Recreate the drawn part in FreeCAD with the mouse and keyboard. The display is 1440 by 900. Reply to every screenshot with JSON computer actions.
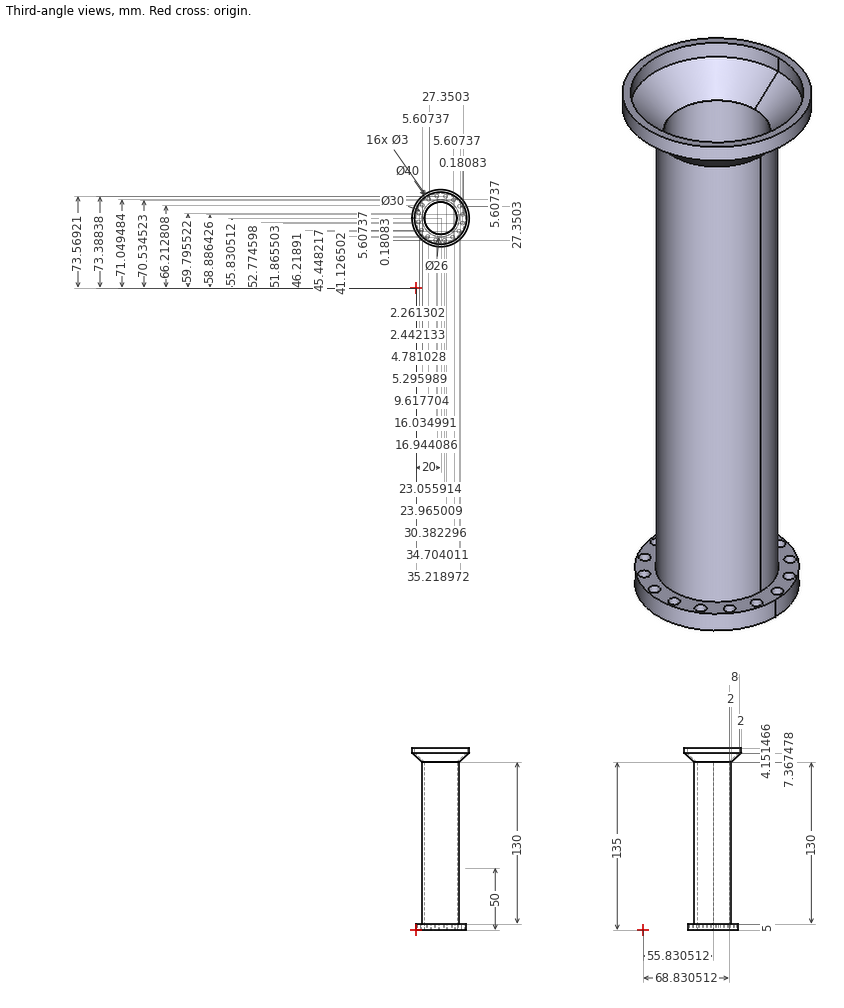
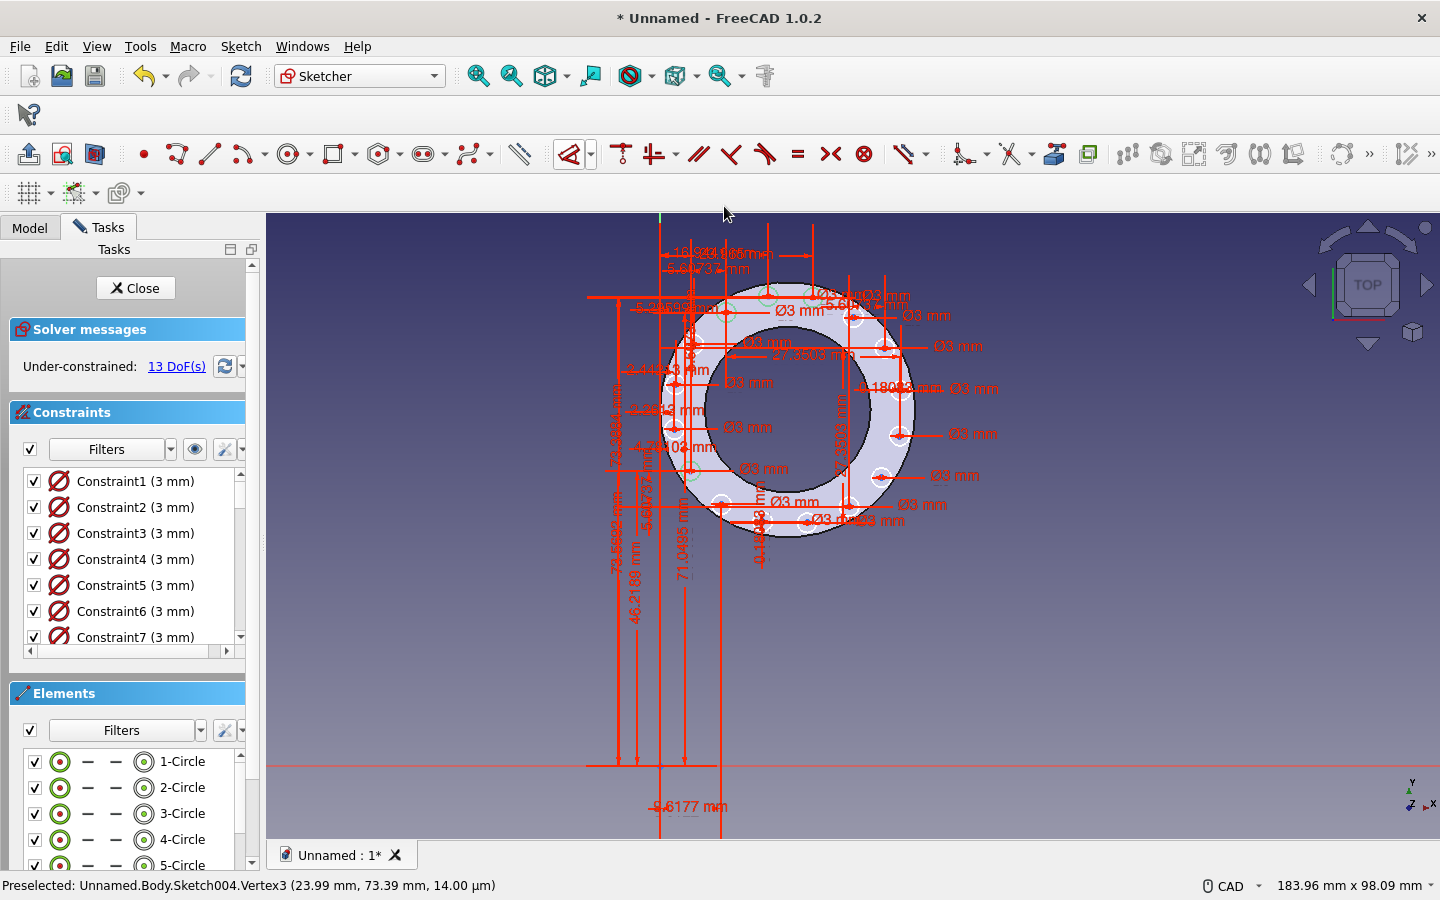
{"action": "left_click", "coordinate": [853, 318]}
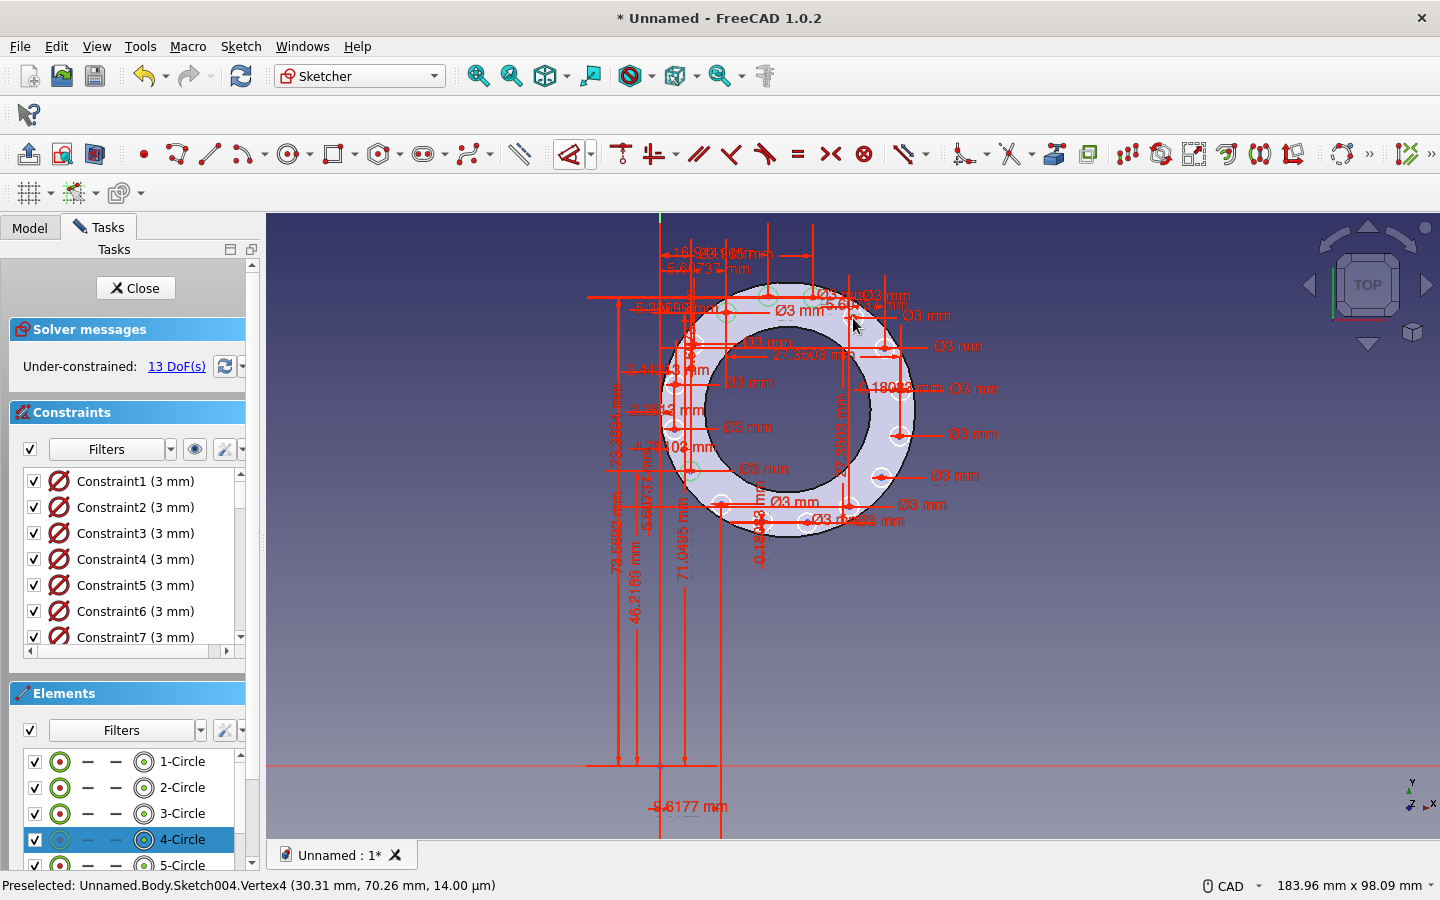
{"action": "key", "text": "l"}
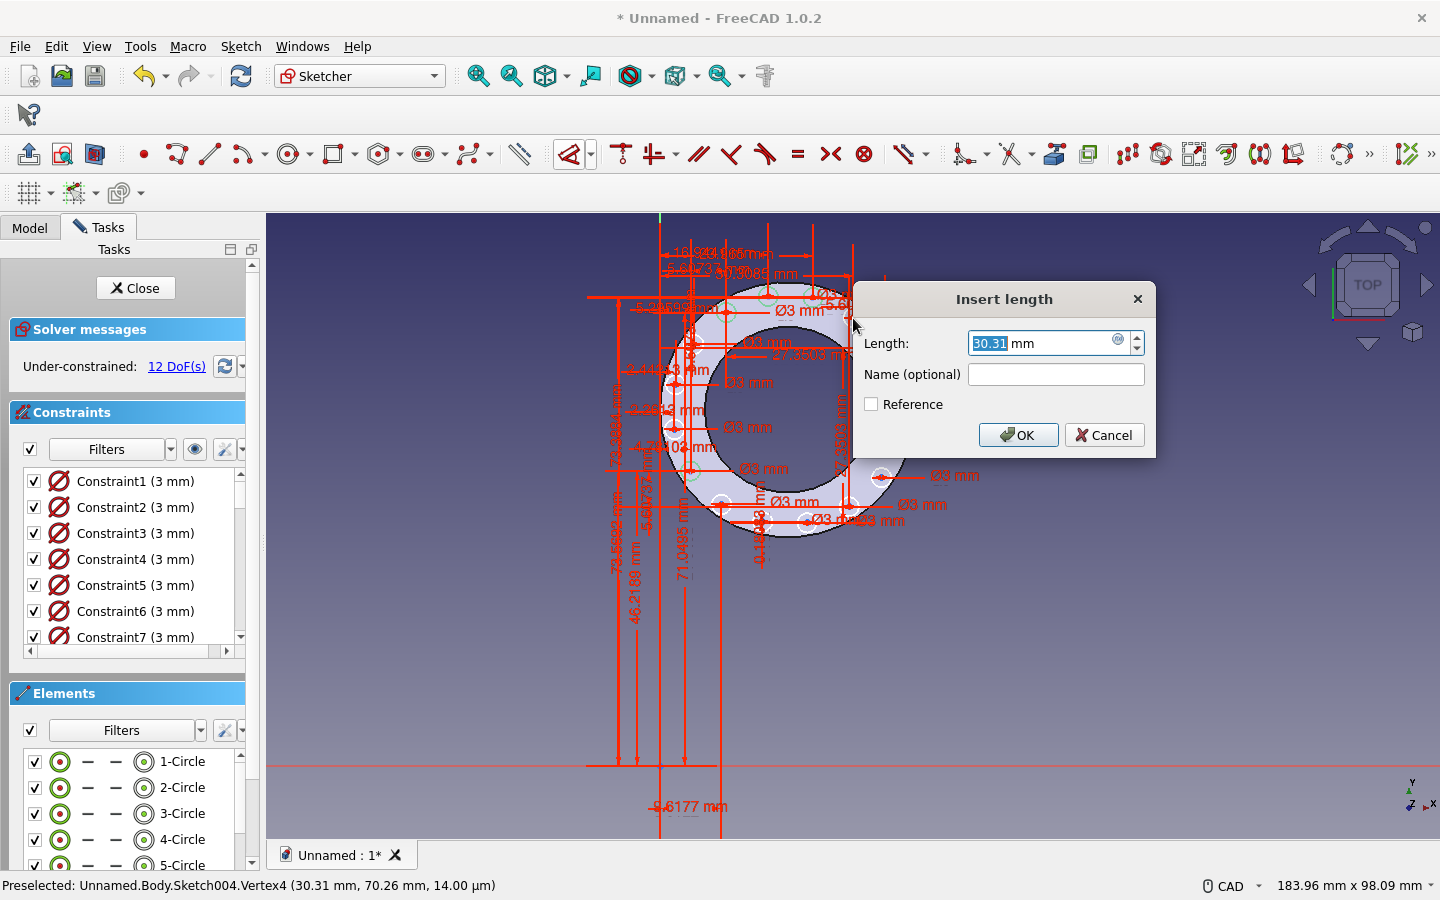
{"action": "type", "text": "30.382296"}
{"action": "key", "text": "Return"}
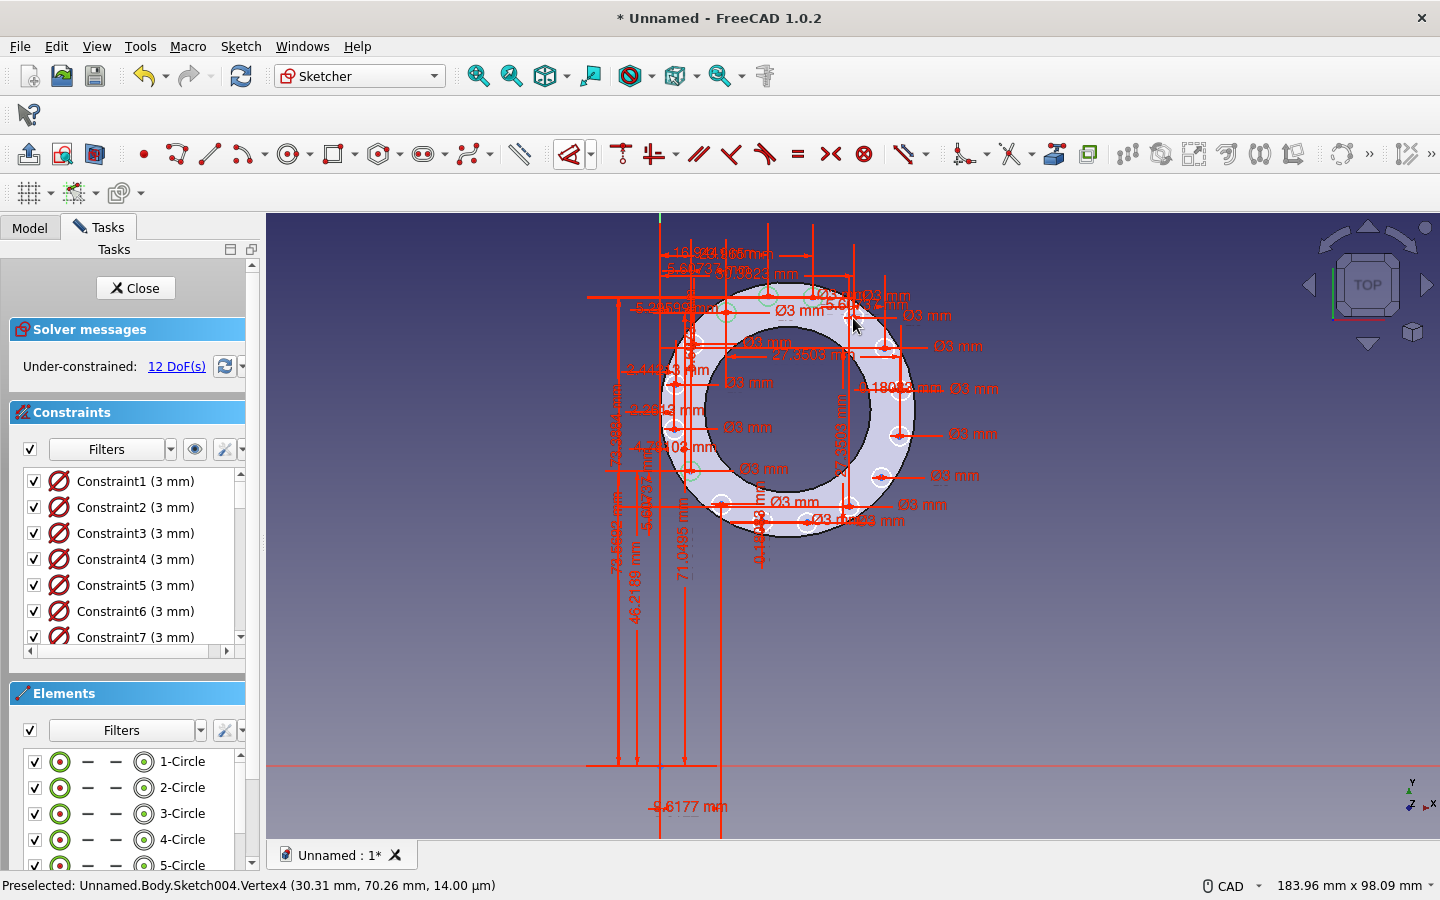
{"action": "left_click", "coordinate": [854, 318]}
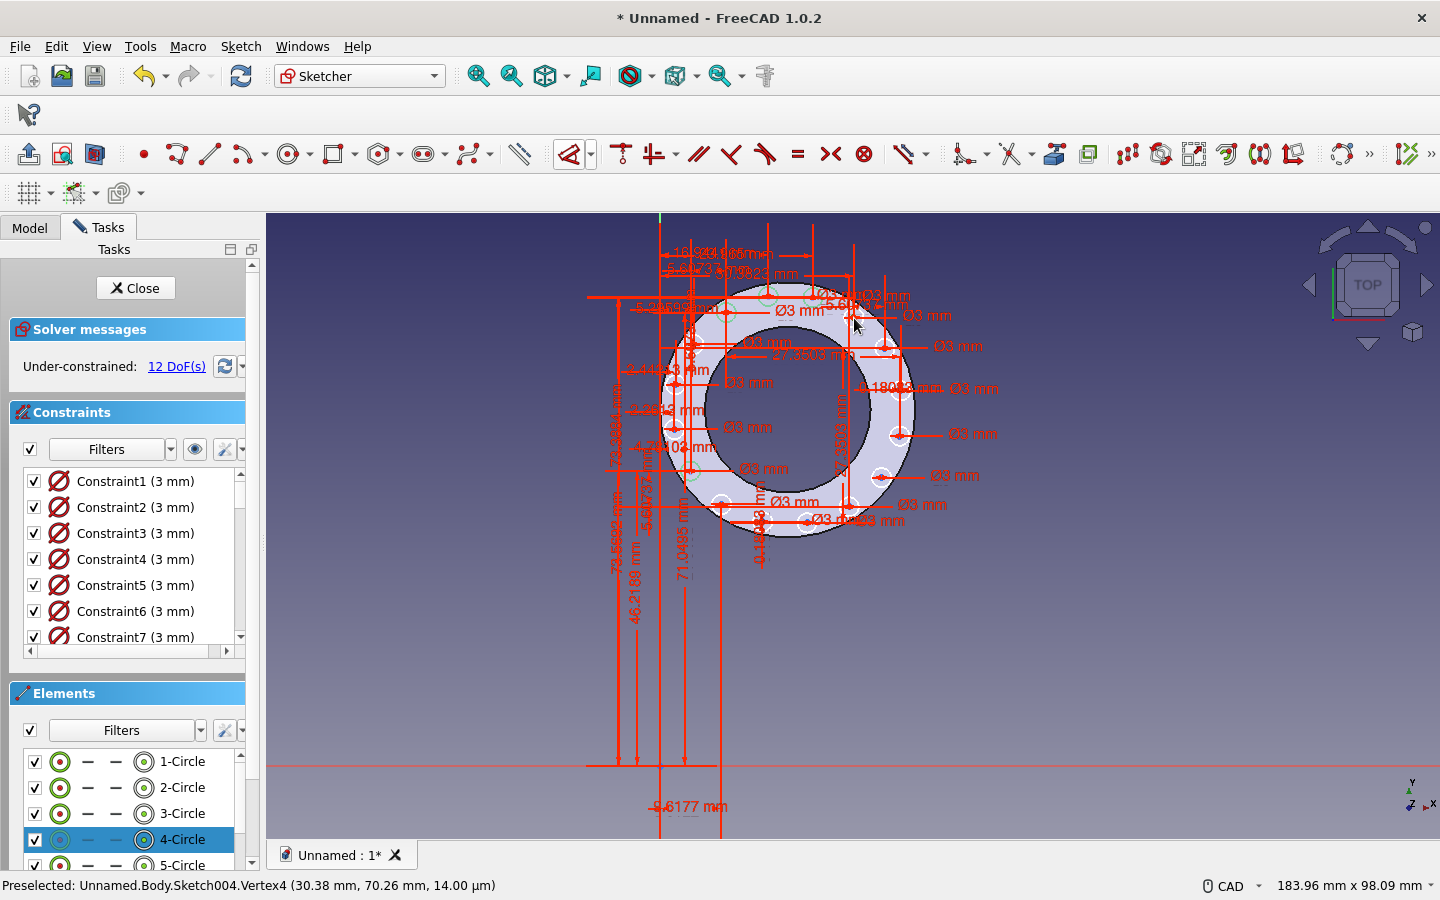
{"action": "key", "text": "i"}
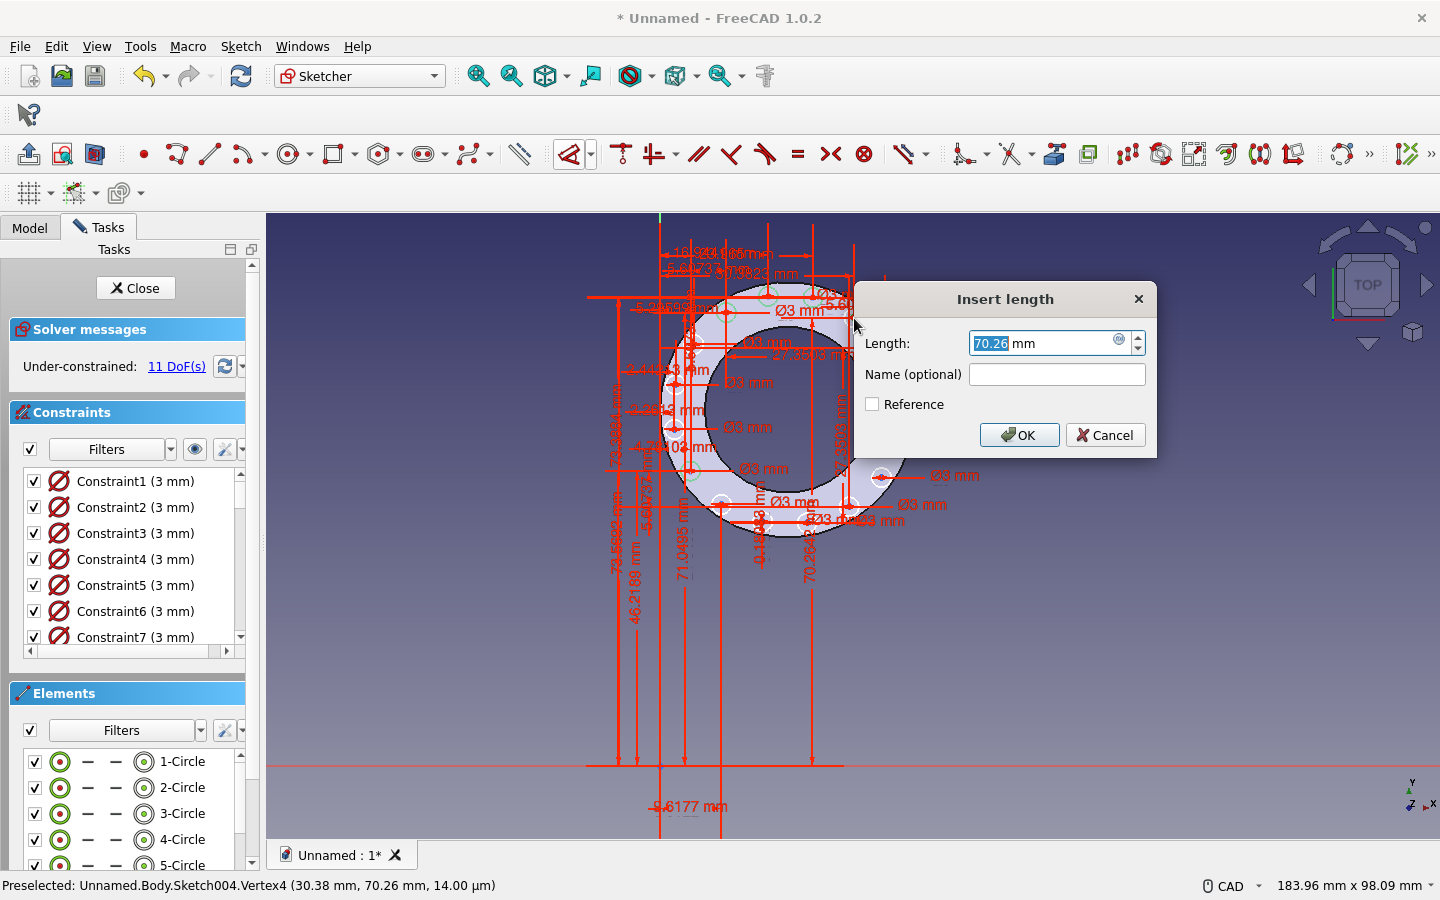
{"action": "type", "text": "70.534523"}
{"action": "key", "text": "Return"}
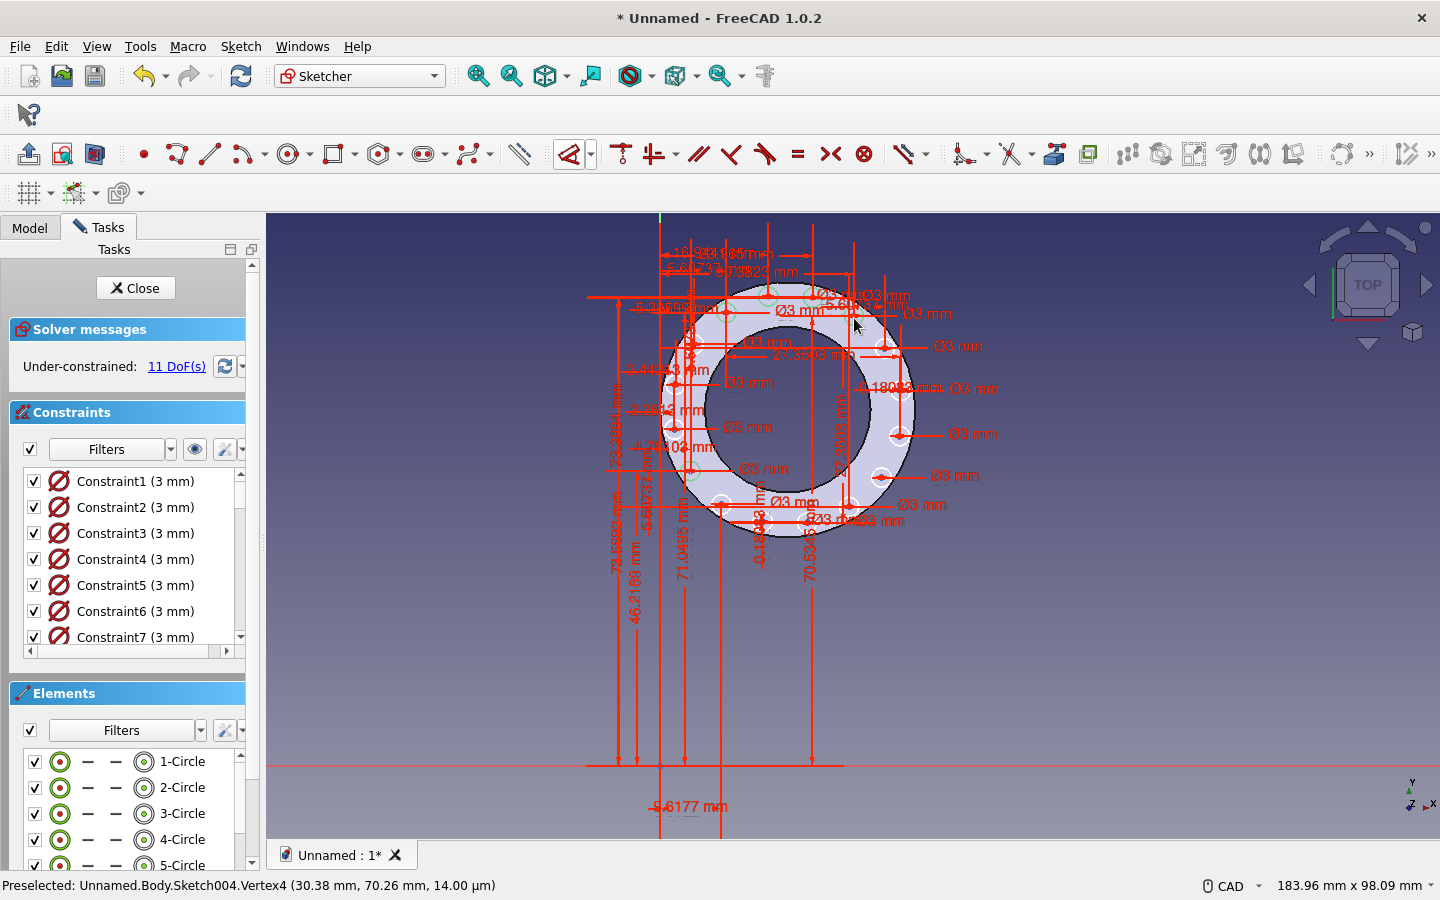
{"action": "left_click", "coordinate": [885, 348]}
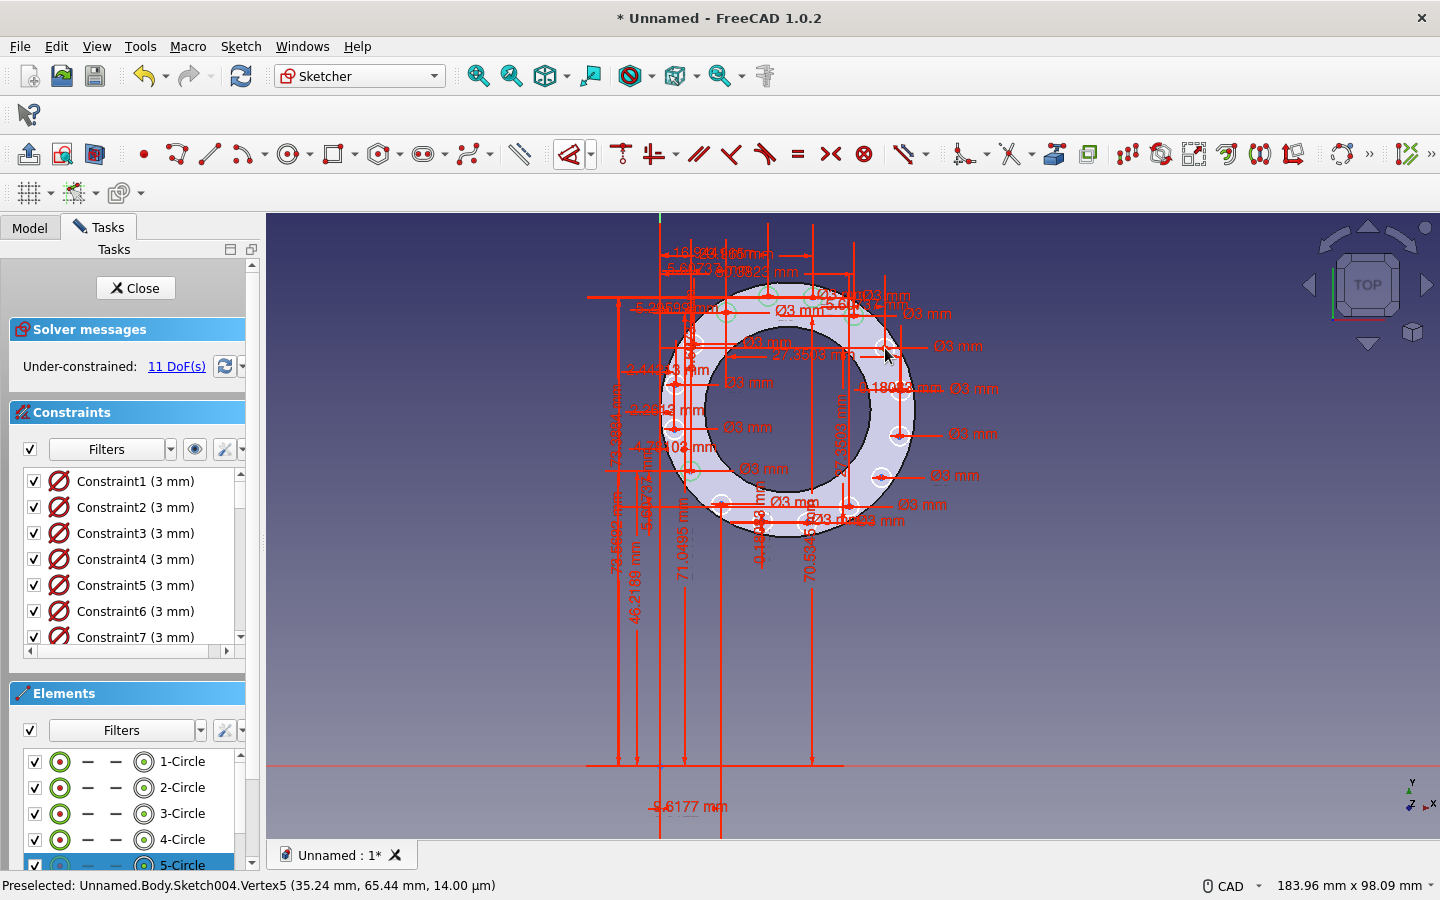
{"action": "left_click", "coordinate": [590, 154]}